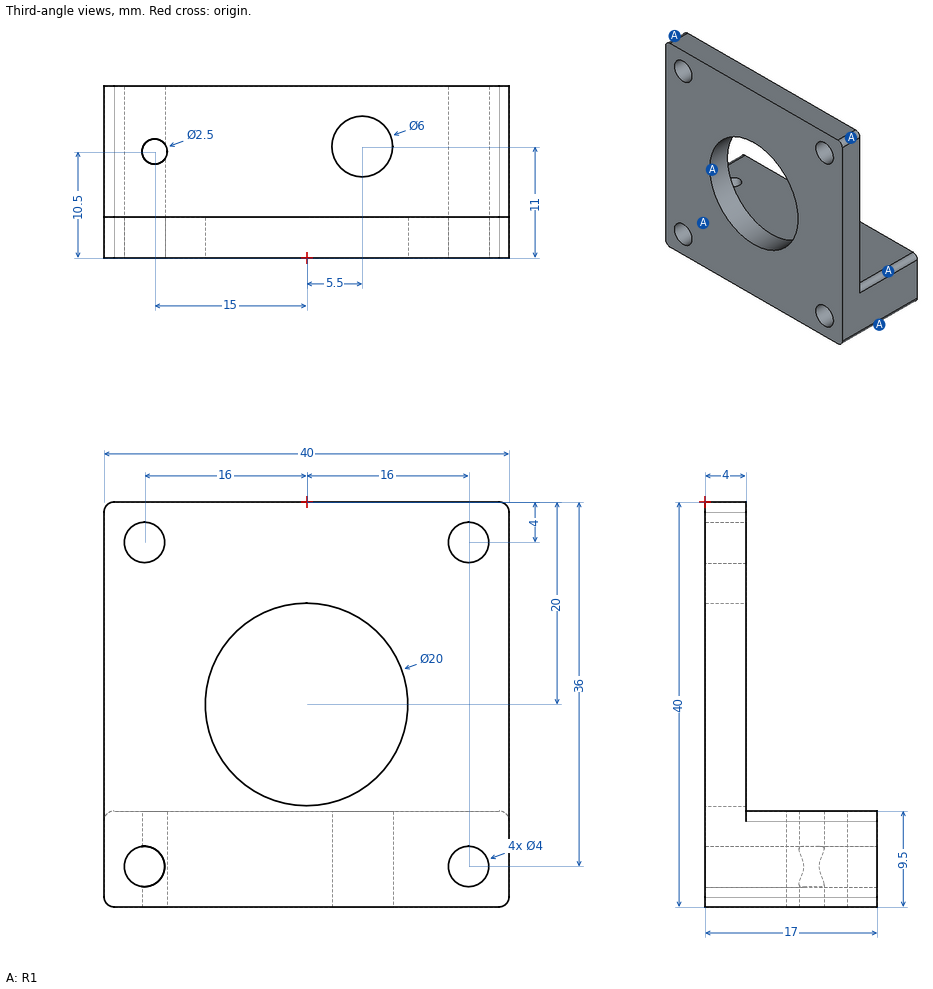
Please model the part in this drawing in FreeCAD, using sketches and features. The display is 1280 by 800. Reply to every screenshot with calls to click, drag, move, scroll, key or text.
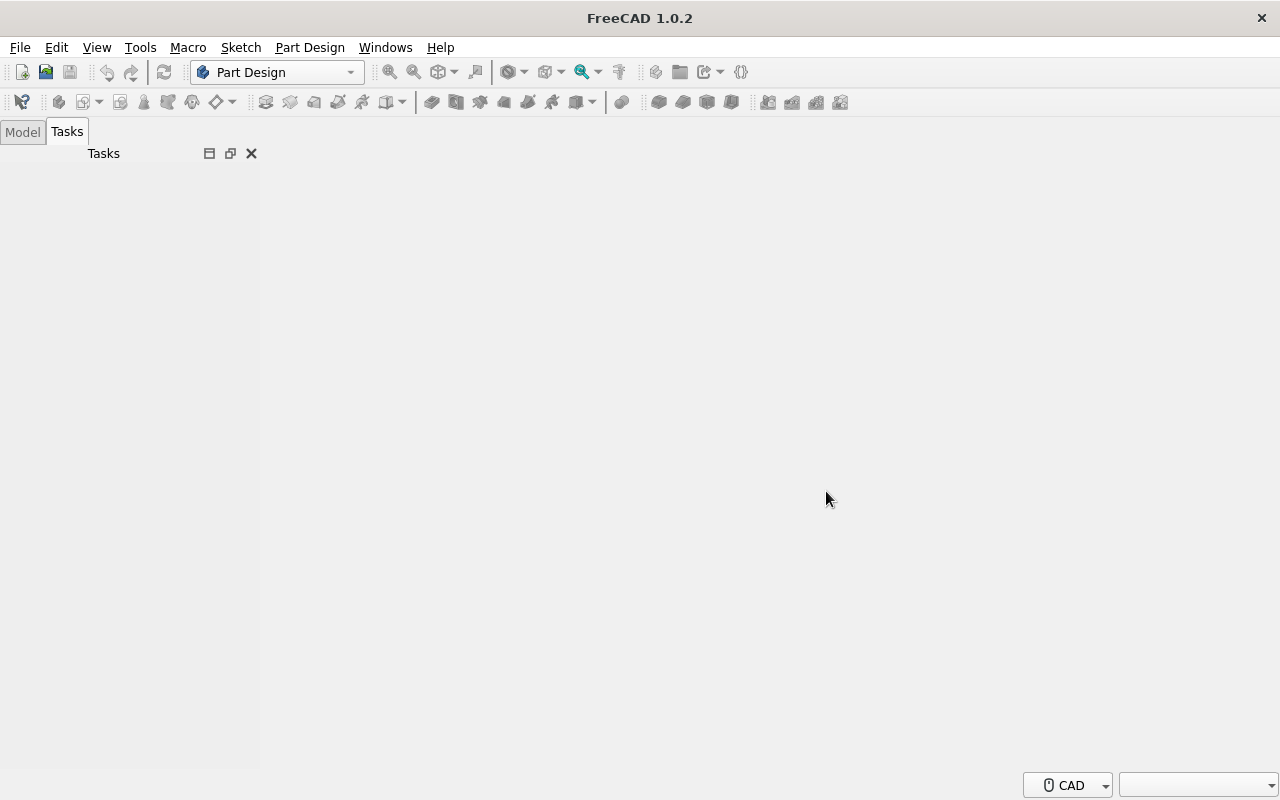
key(ctrl+n)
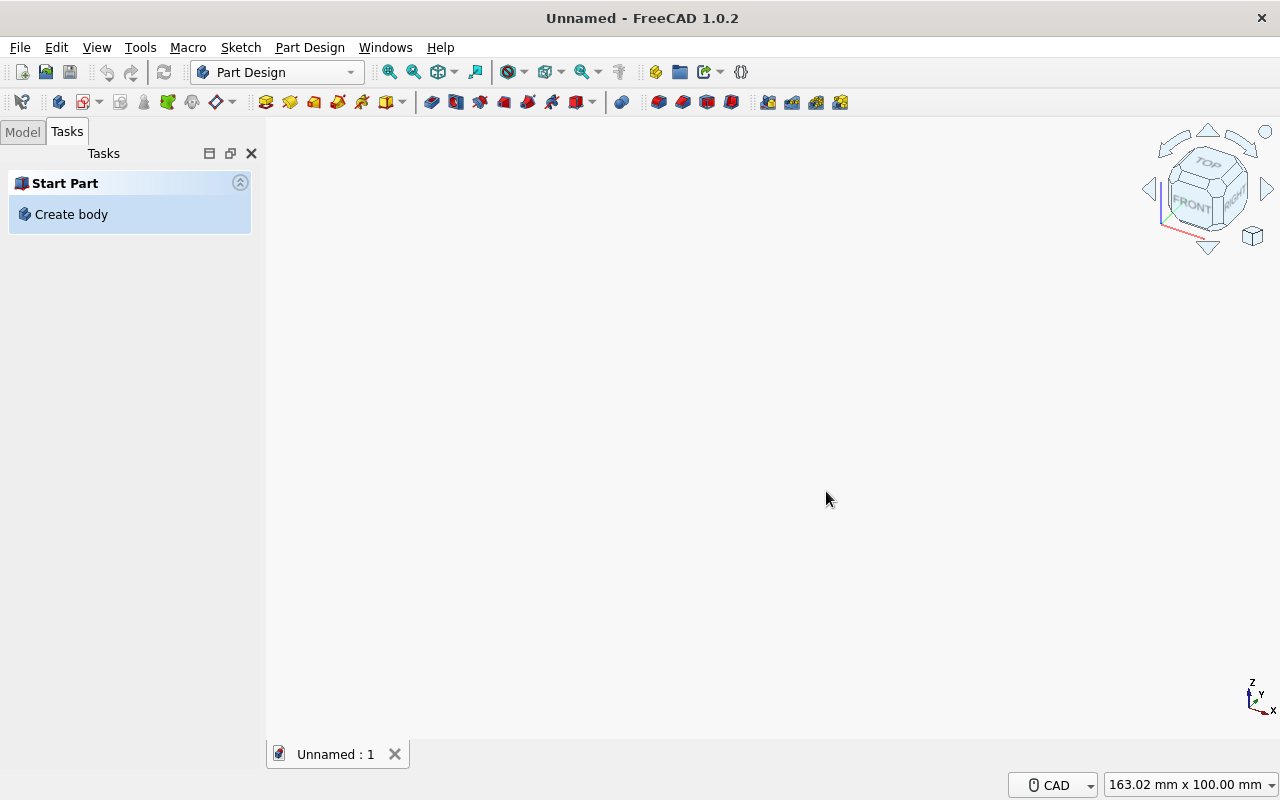
click(84, 102)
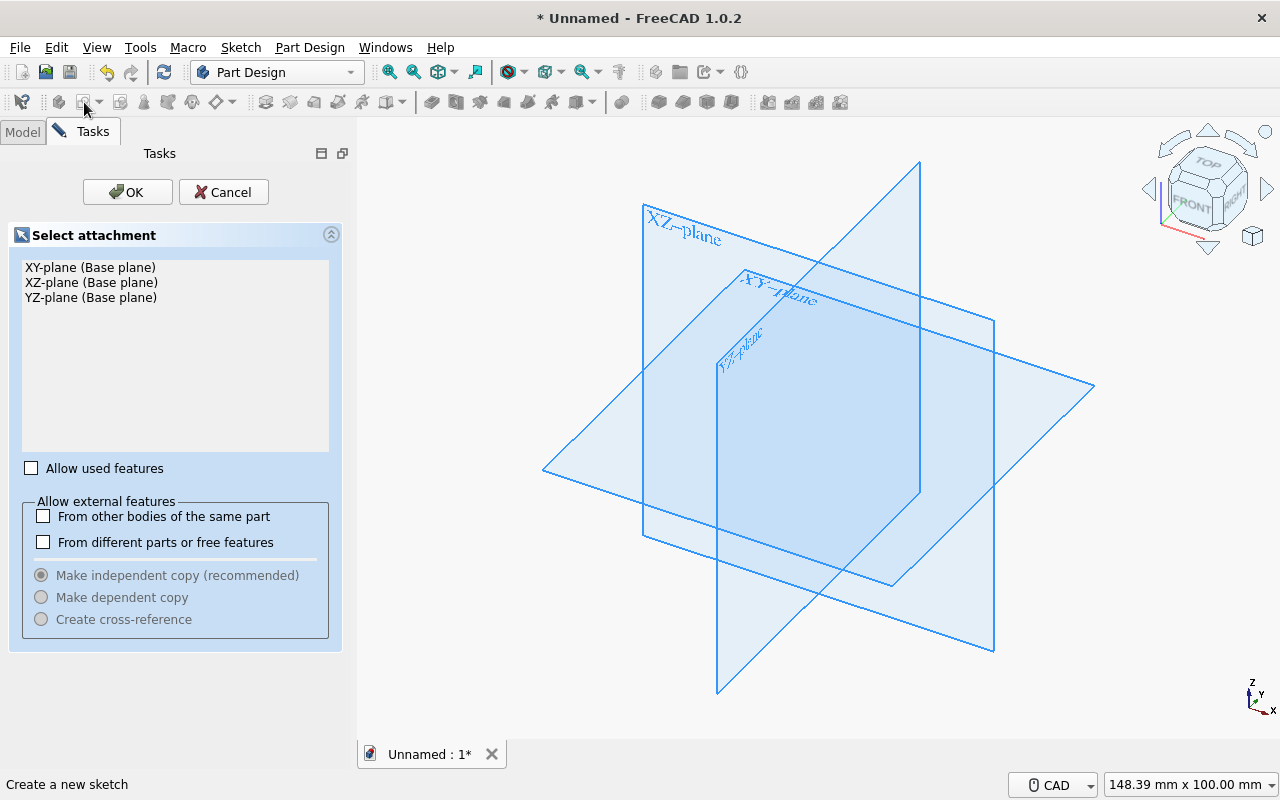
click(82, 298)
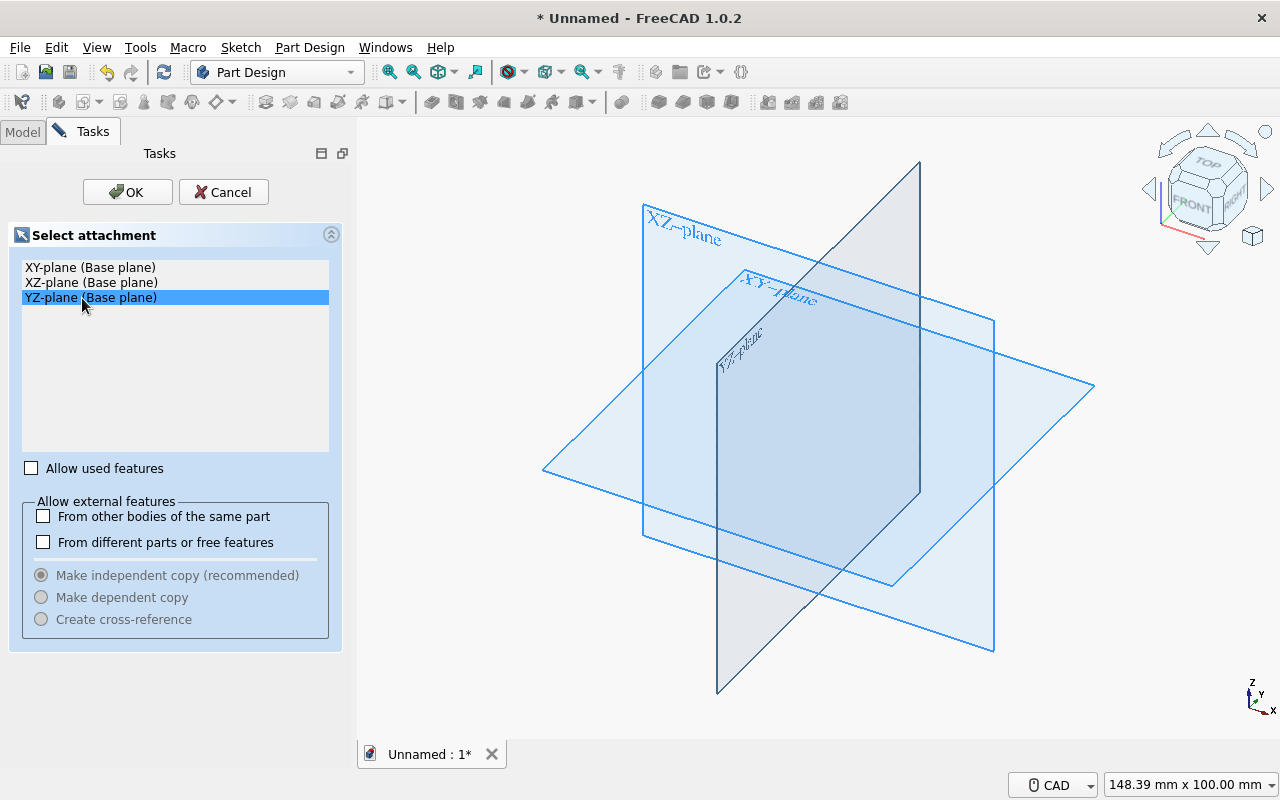
click(128, 192)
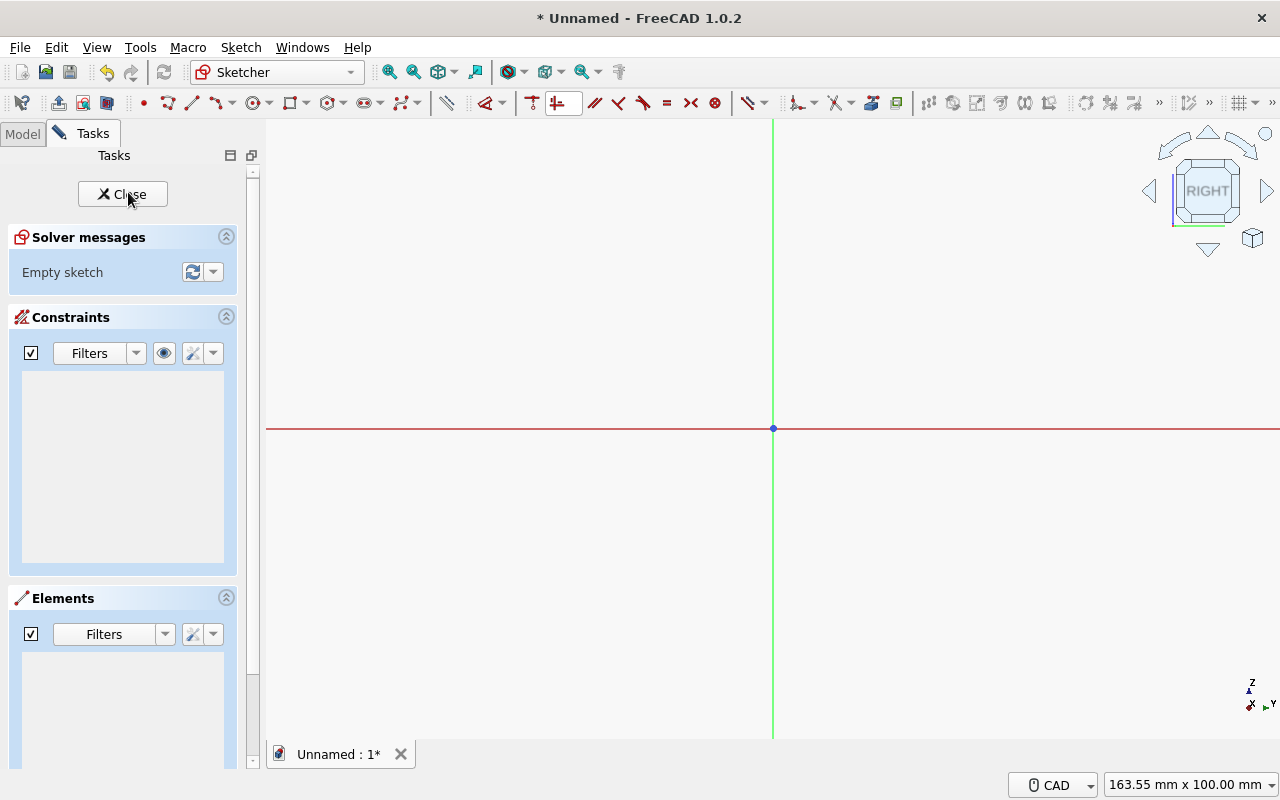
scroll(1072, 711, up, 2)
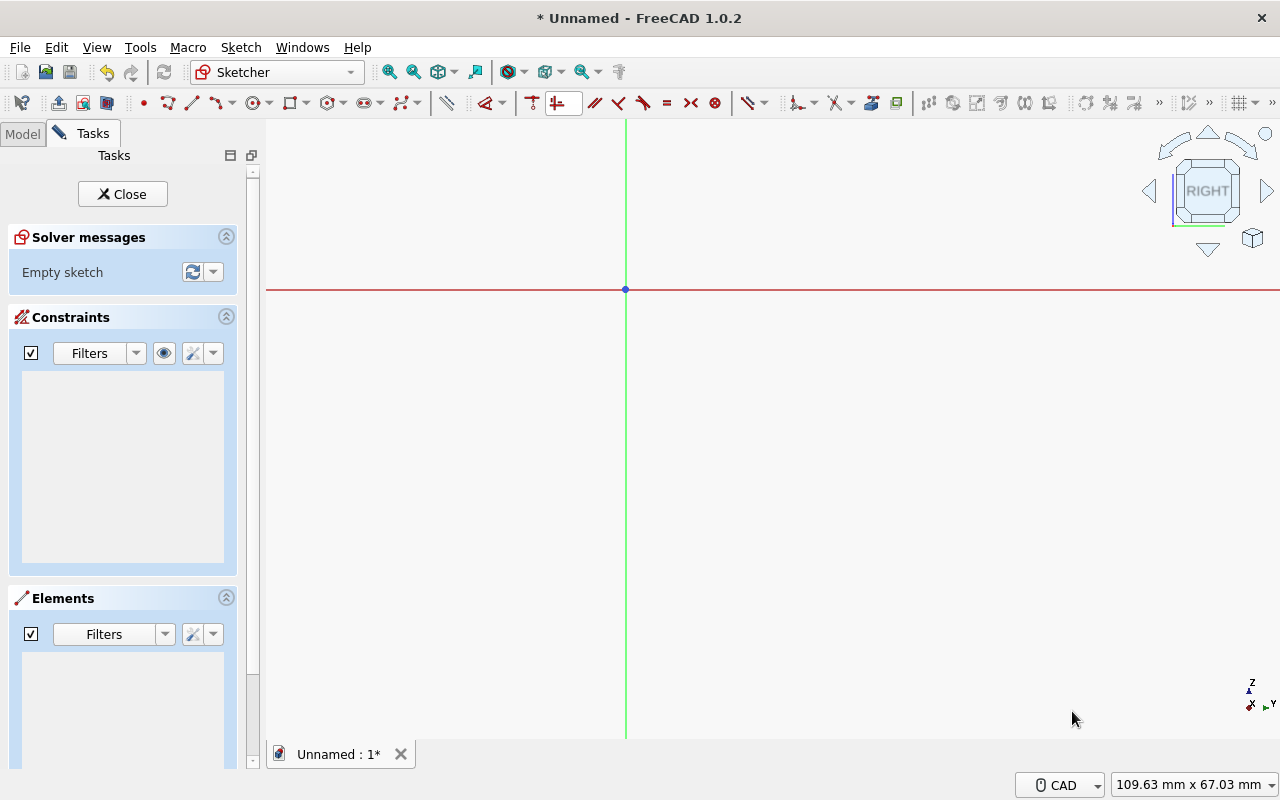
key(g)
key(m)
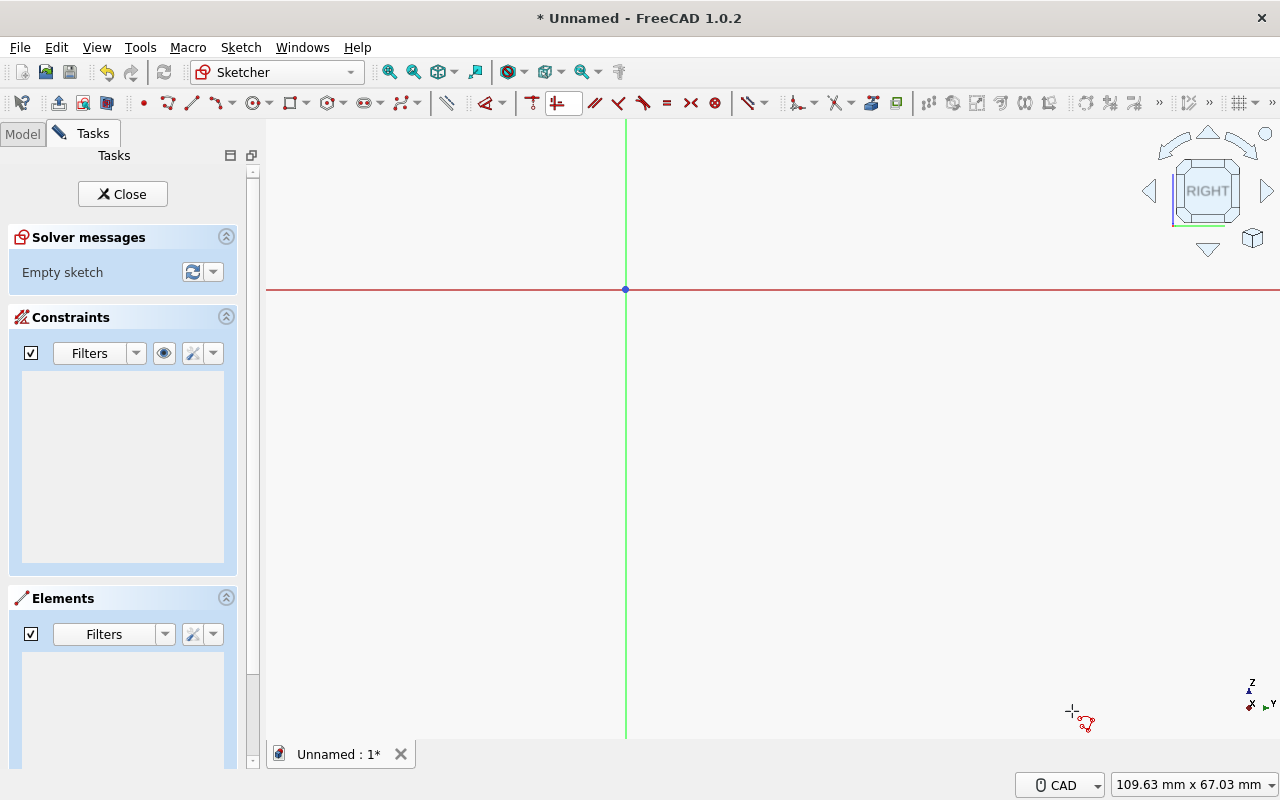
click(626, 290)
click(635, 660)
click(783, 660)
click(783, 572)
click(663, 572)
click(663, 299)
click(626, 290)
key(Escape)
key(Escape)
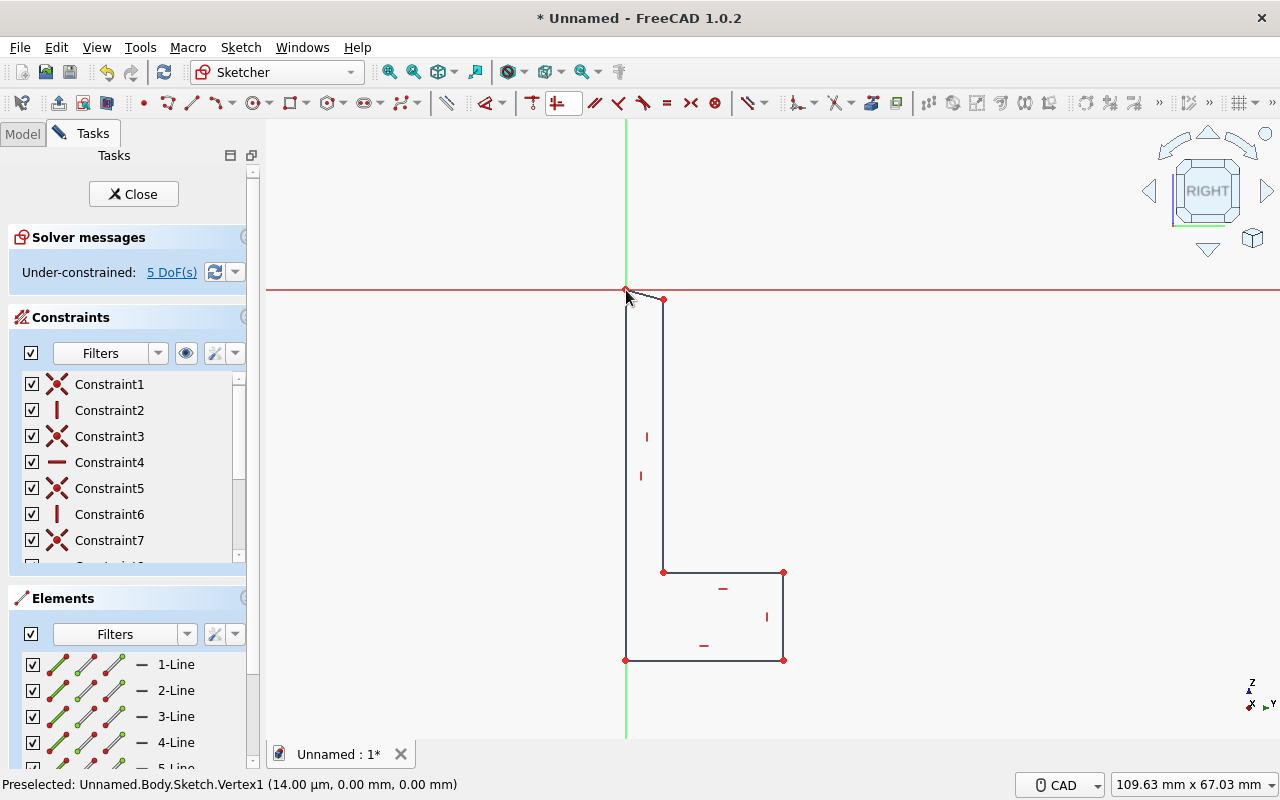
scroll(637, 293, up, 2)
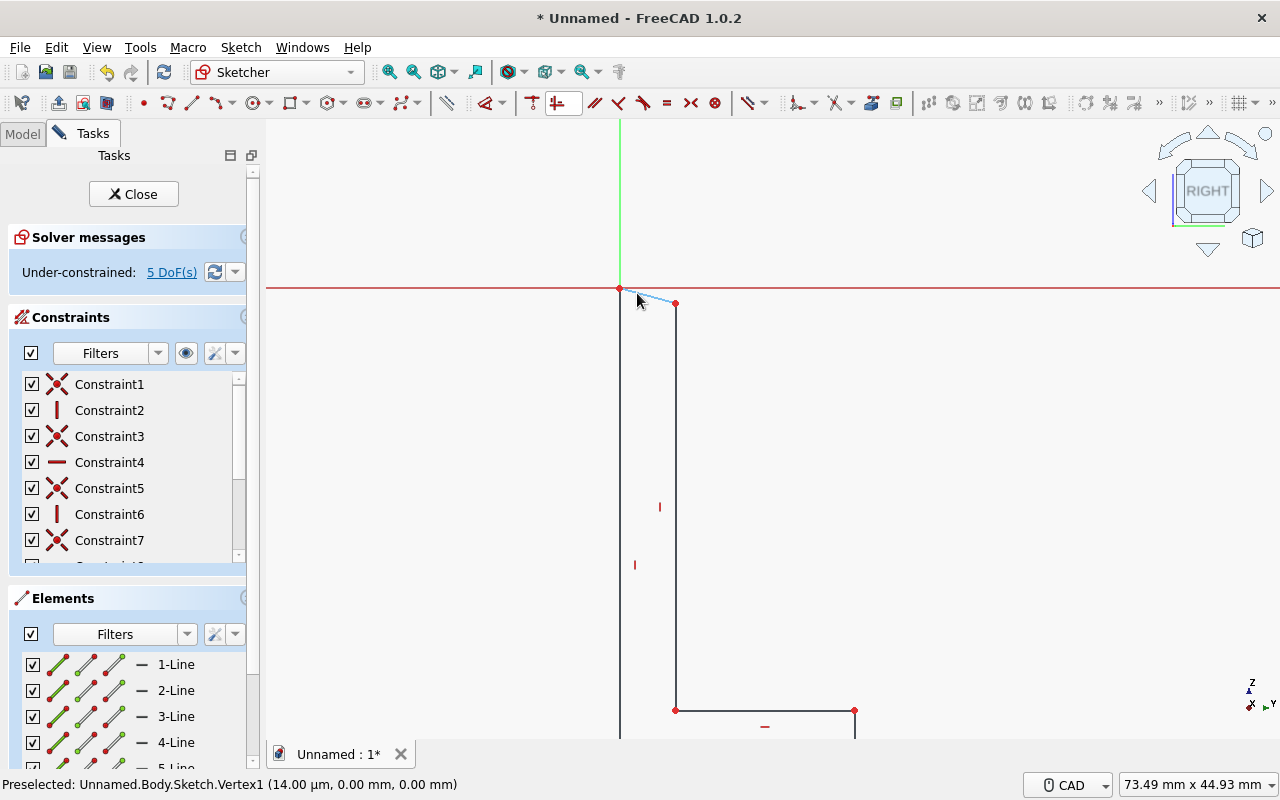
click(637, 293)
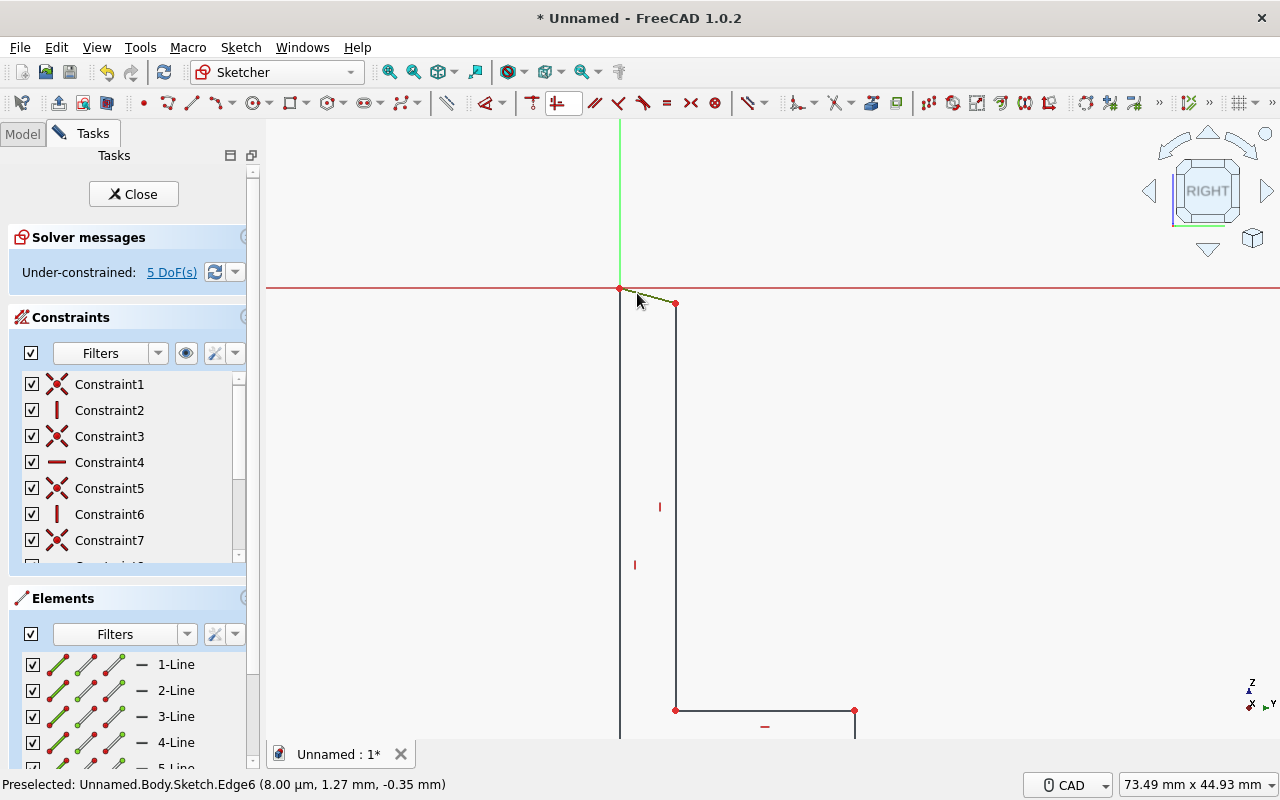
click(576, 104)